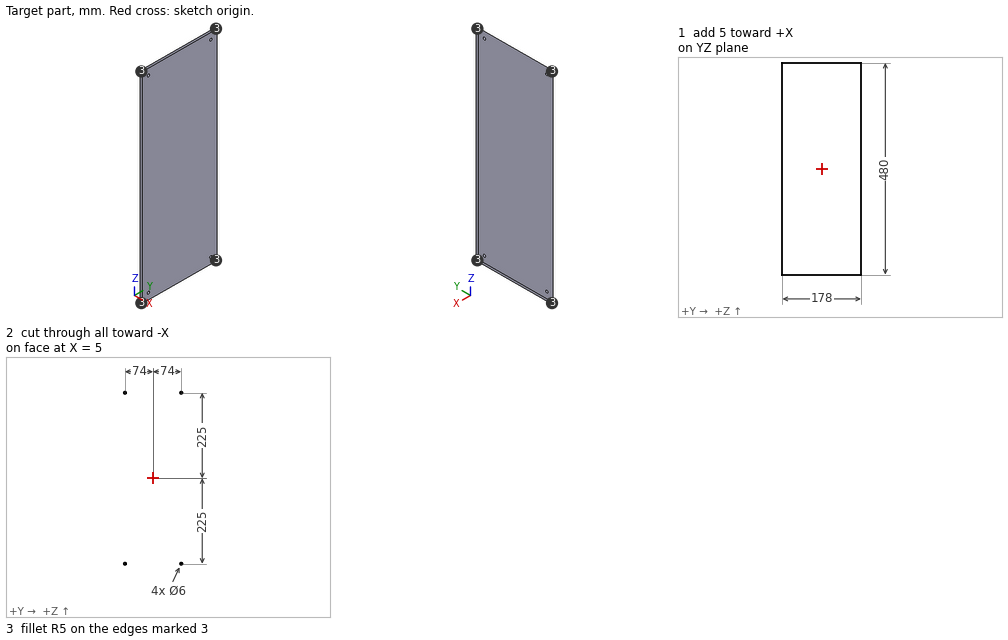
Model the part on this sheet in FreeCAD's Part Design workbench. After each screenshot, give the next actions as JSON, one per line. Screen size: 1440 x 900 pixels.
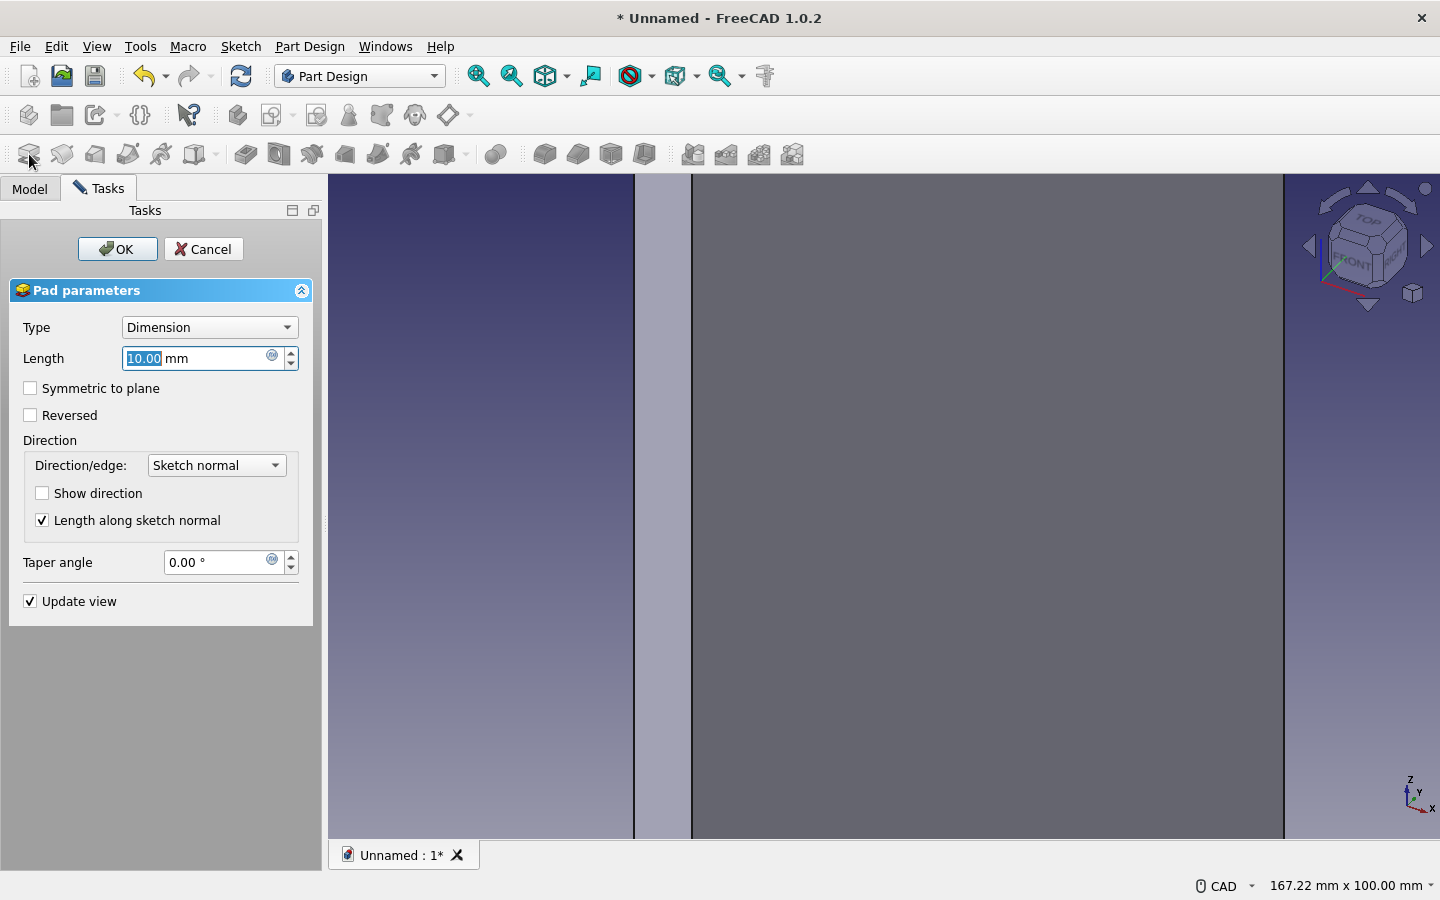
{"action": "type", "text": "5"}
{"action": "key", "text": "Tab"}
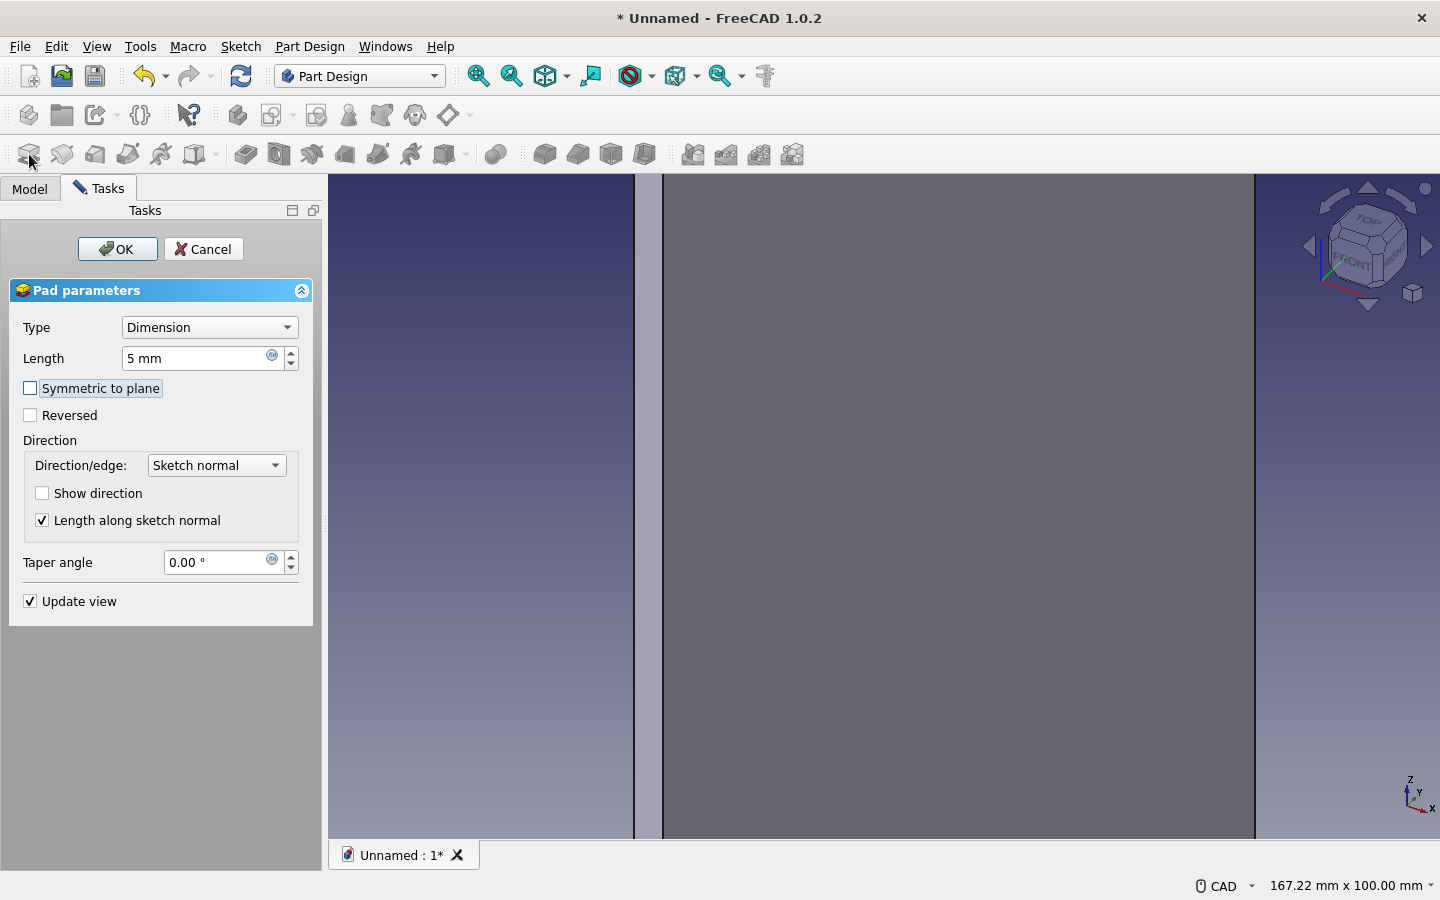
{"action": "left_click", "coordinate": [118, 249]}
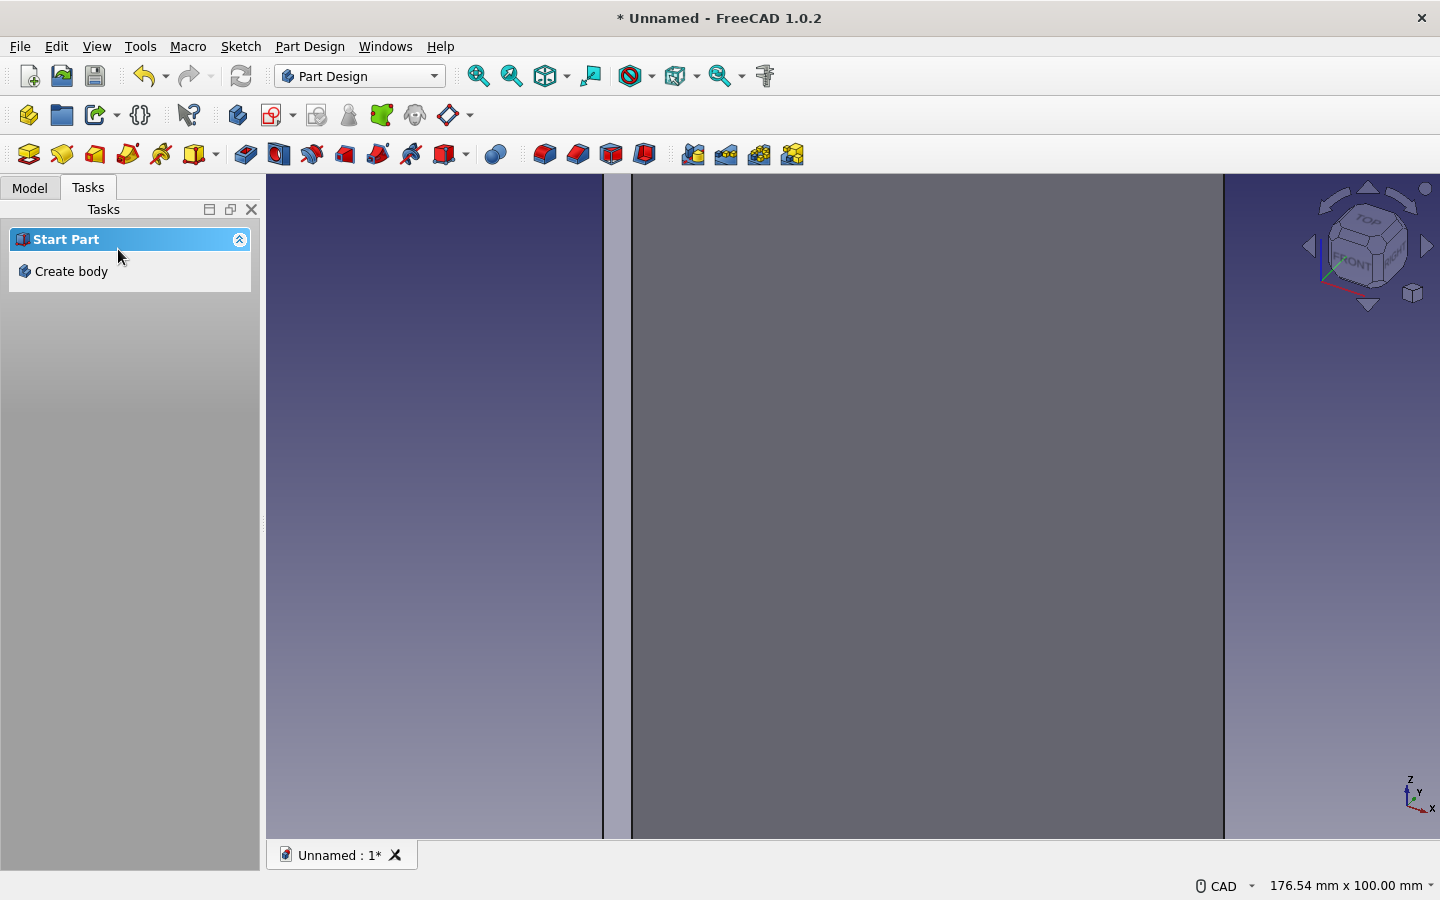
{"action": "left_click", "coordinate": [479, 76]}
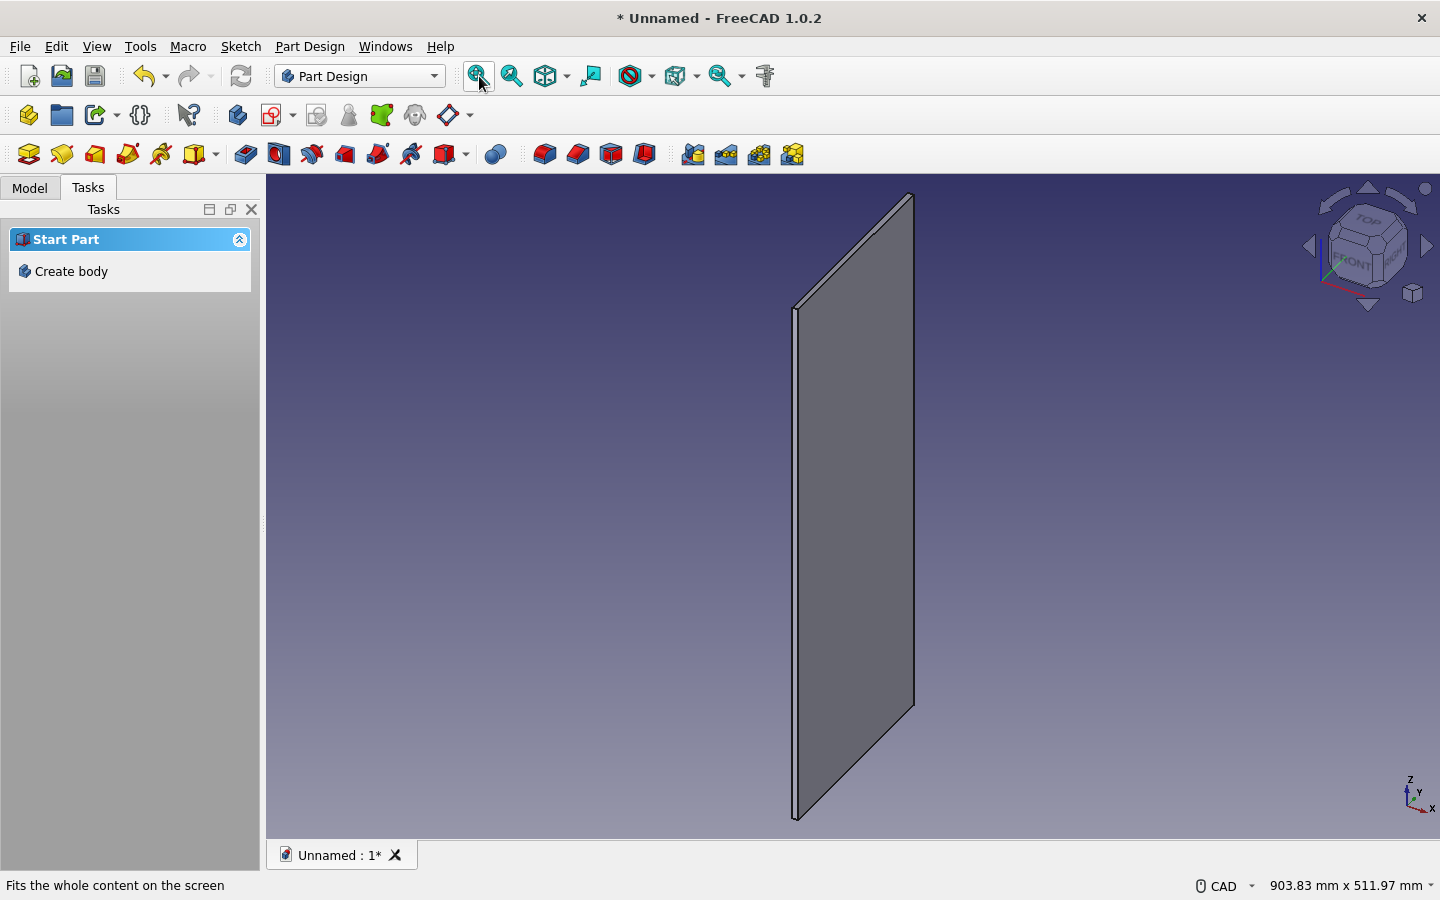
{"action": "left_click", "coordinate": [856, 652]}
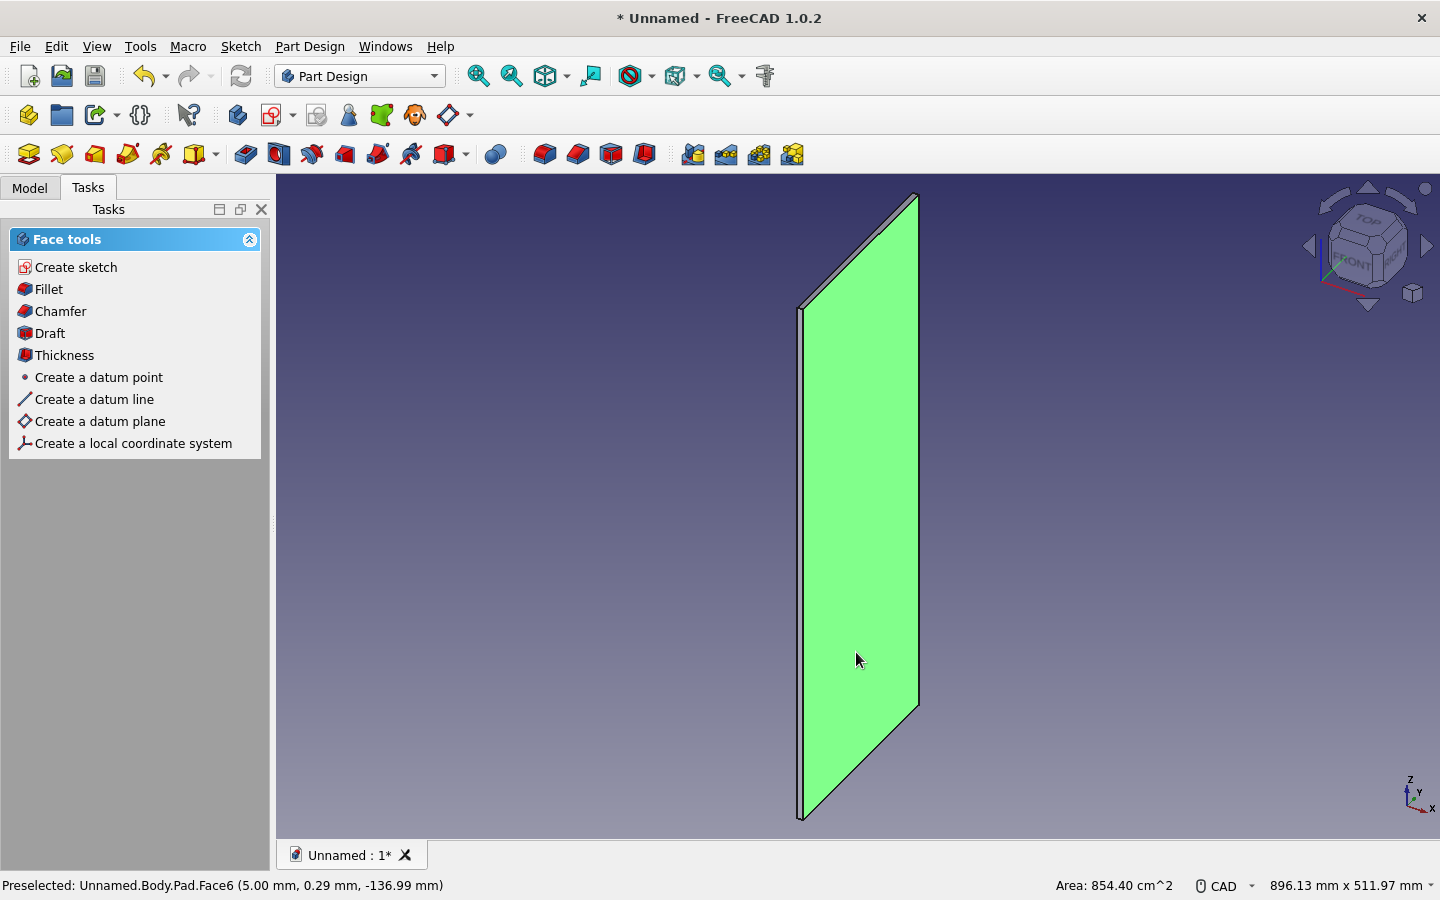
{"action": "left_click", "coordinate": [270, 116]}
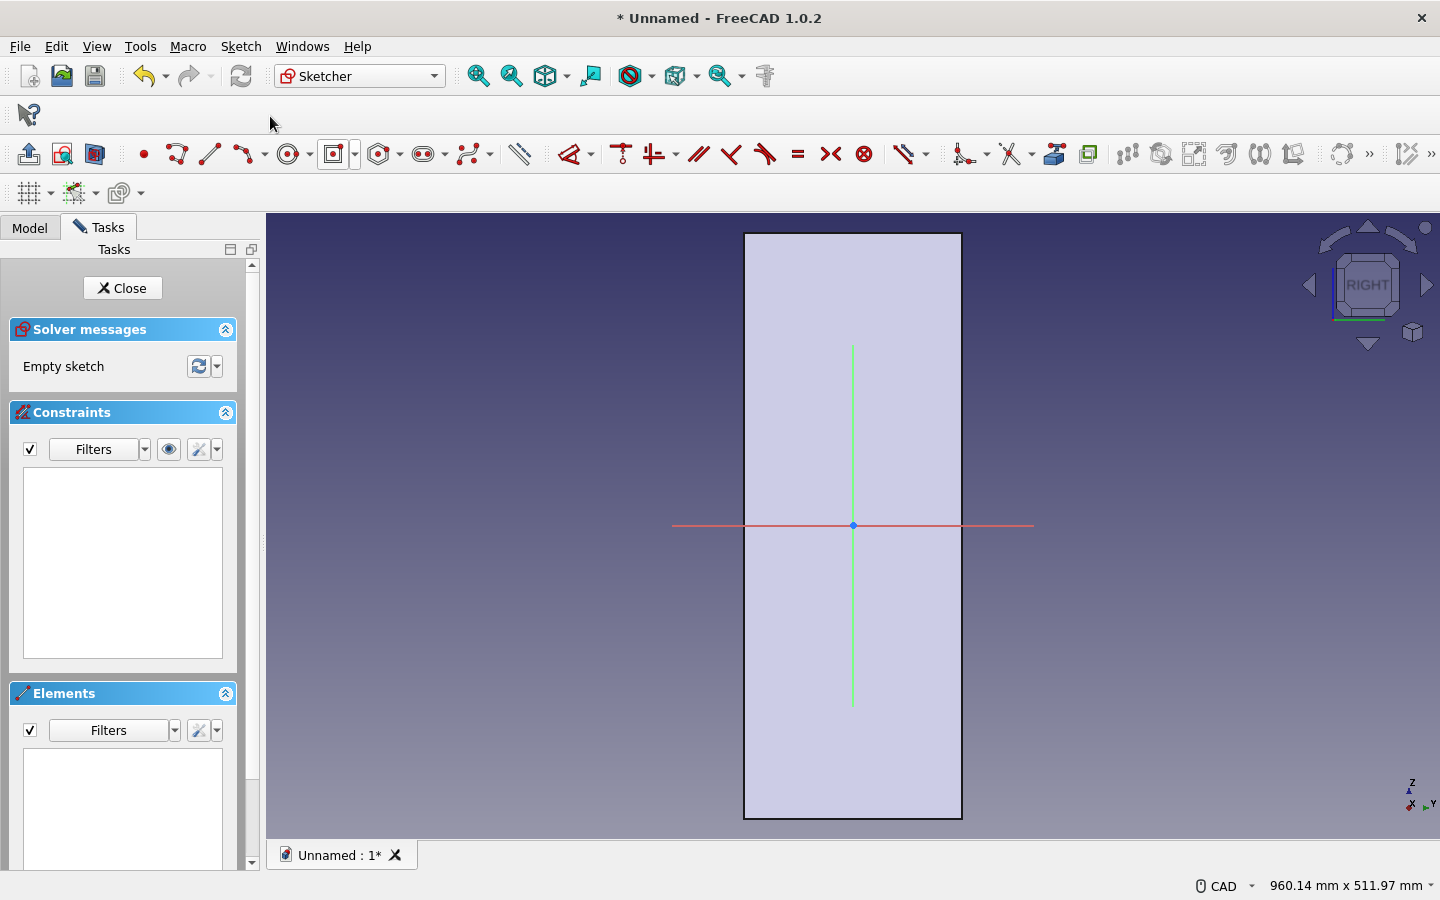
{"action": "scroll", "coordinate": [645, 526], "scroll_direction": "down", "scroll_amount": 2}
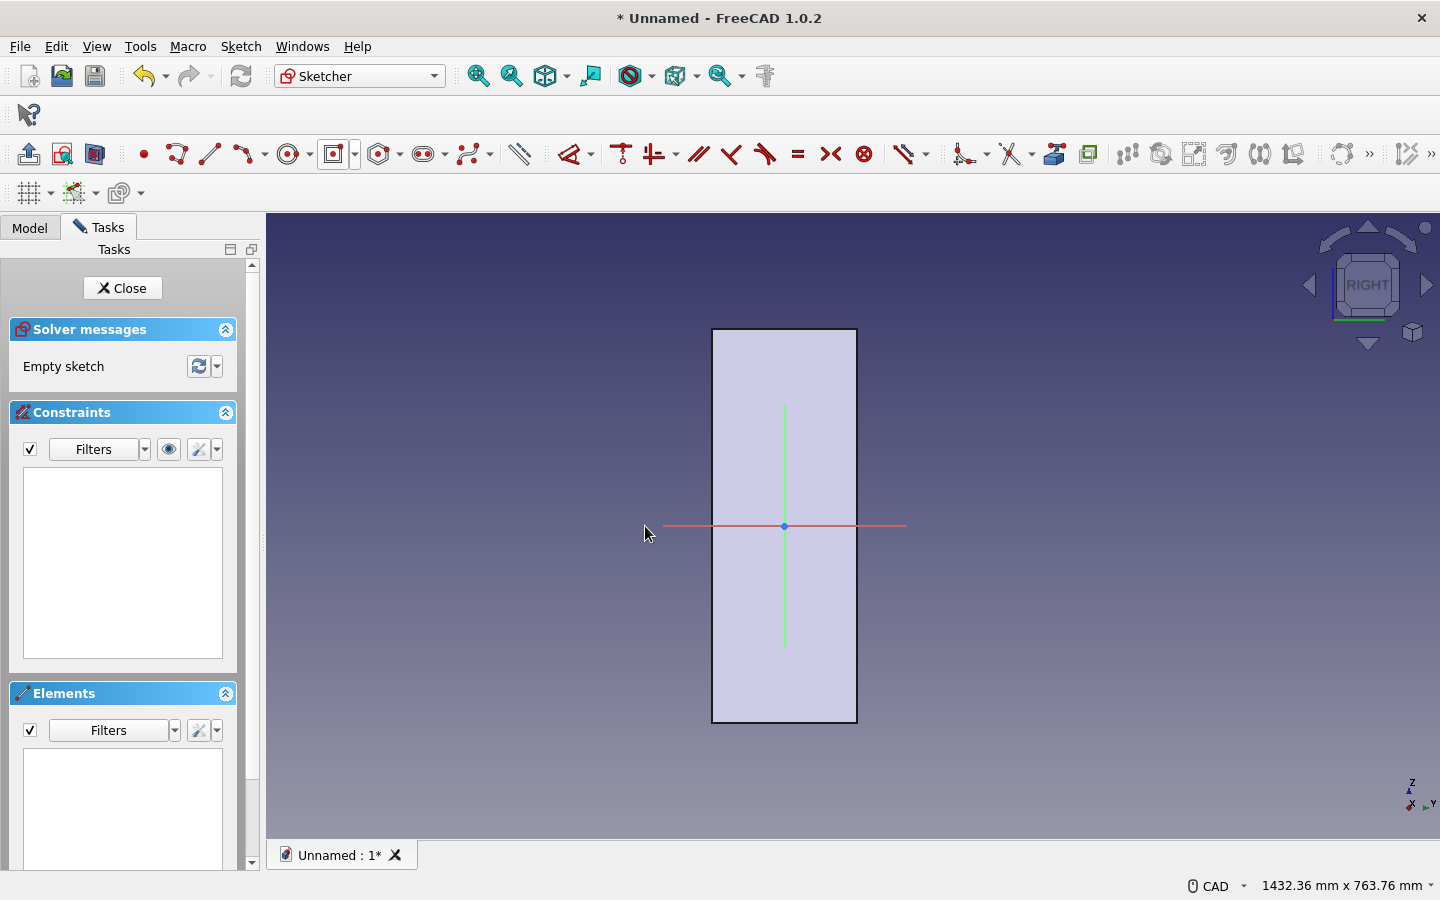
{"action": "left_click", "coordinate": [288, 154]}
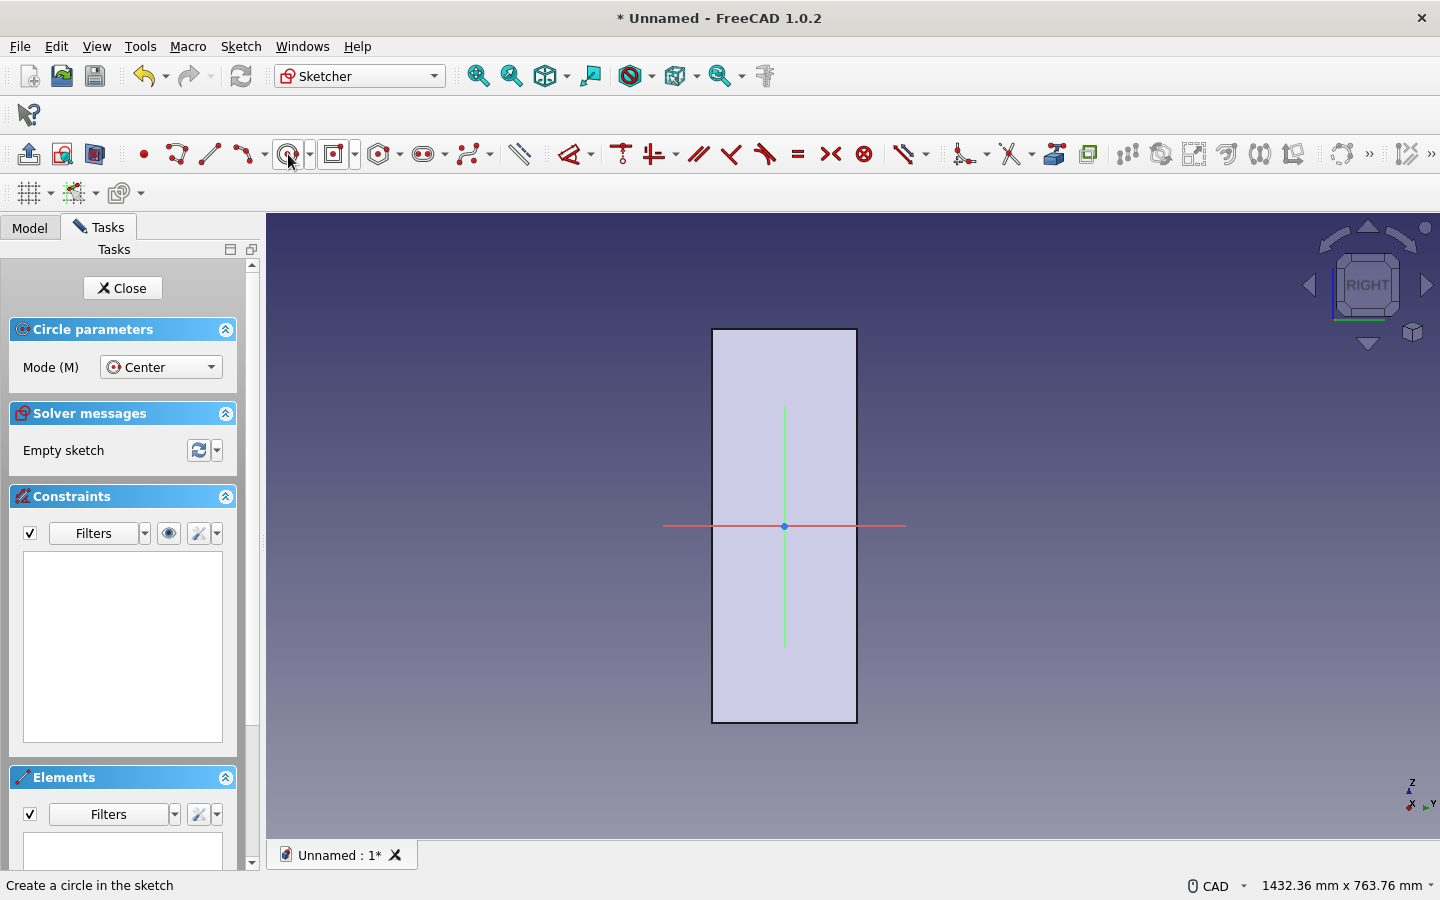
{"action": "scroll", "coordinate": [845, 342], "scroll_direction": "up", "scroll_amount": 12}